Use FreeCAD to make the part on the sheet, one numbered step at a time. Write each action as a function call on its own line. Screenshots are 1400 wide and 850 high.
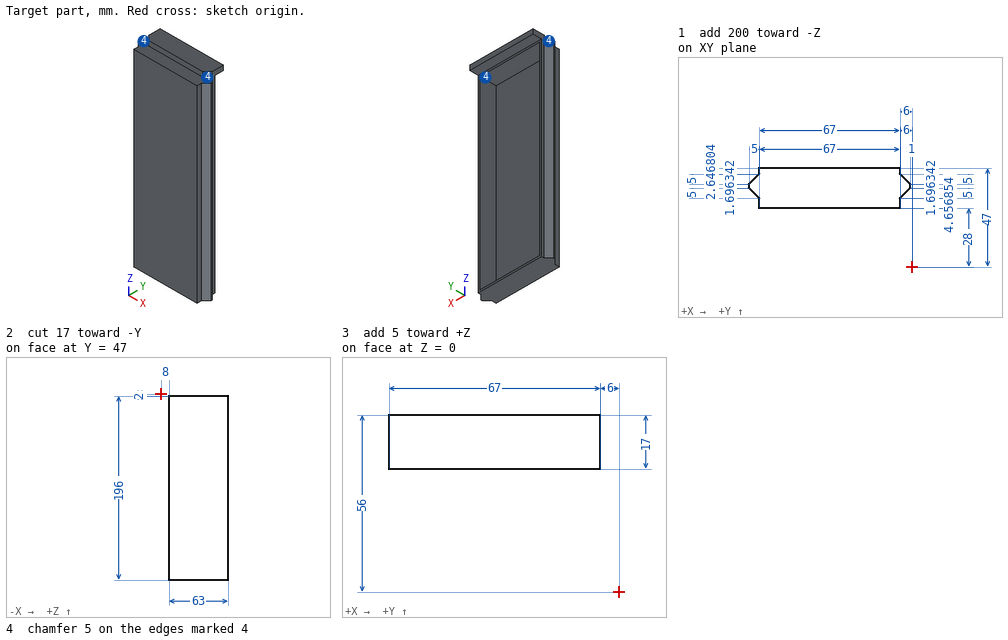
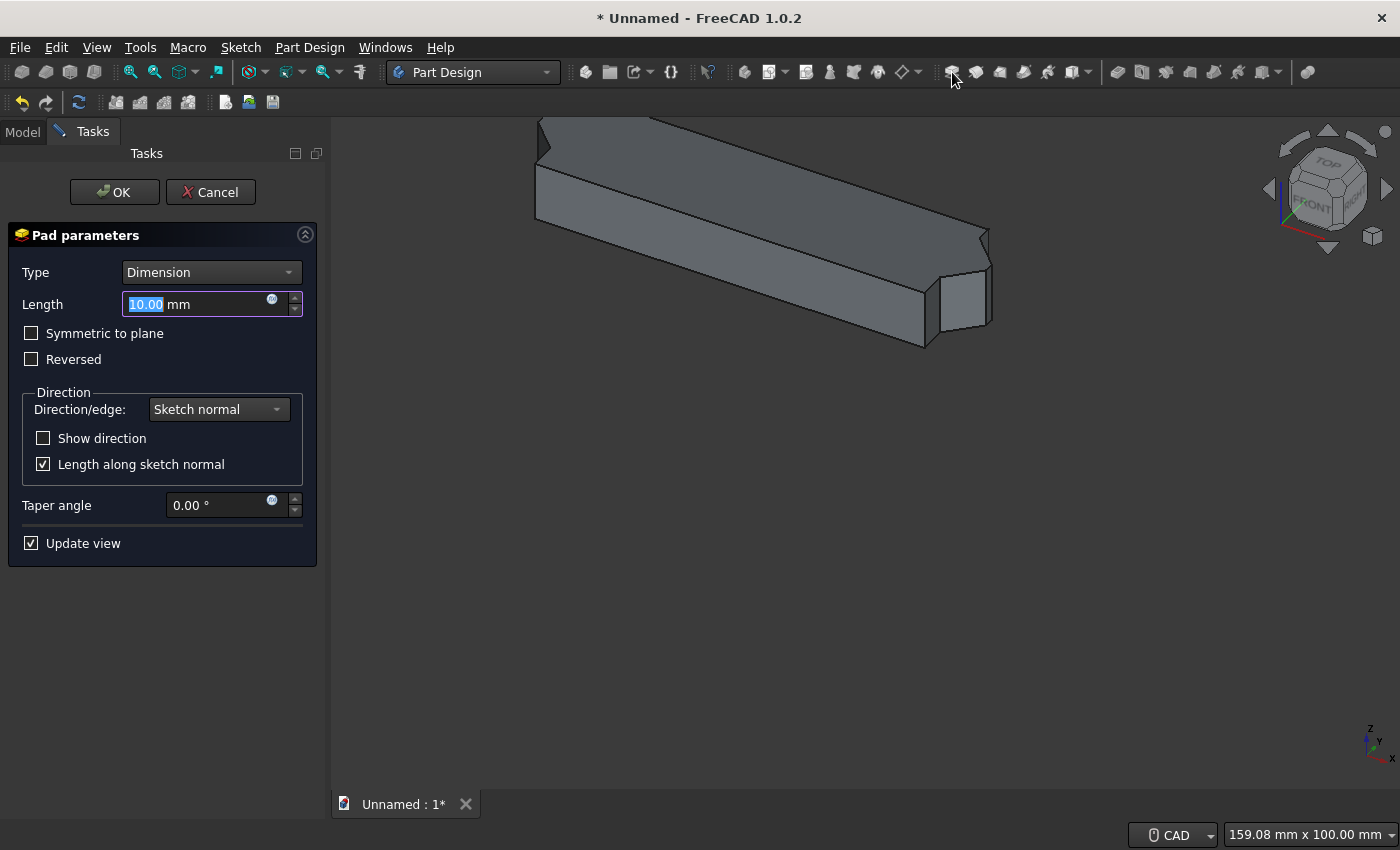
text(200)
key(Tab)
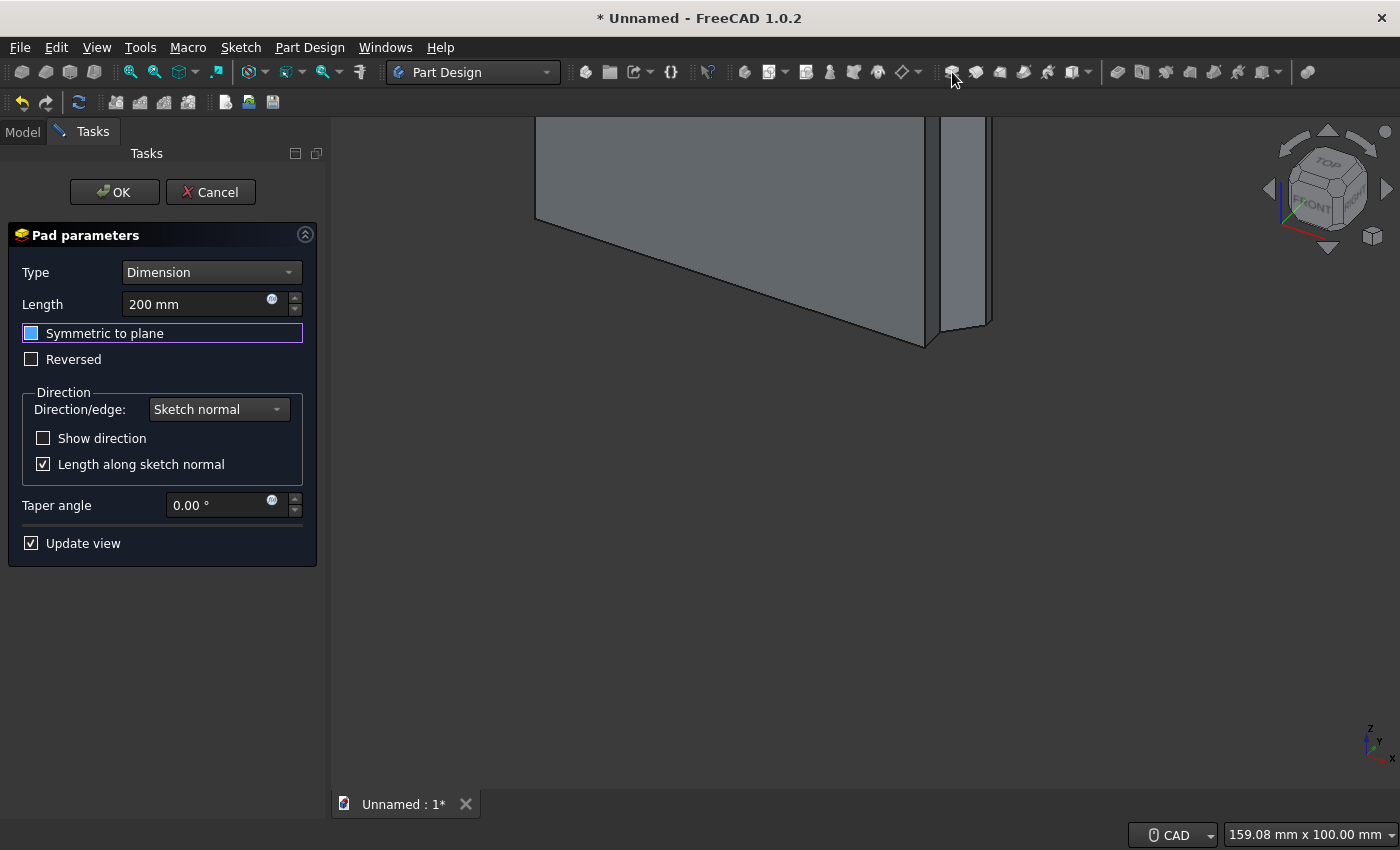
click(30, 359)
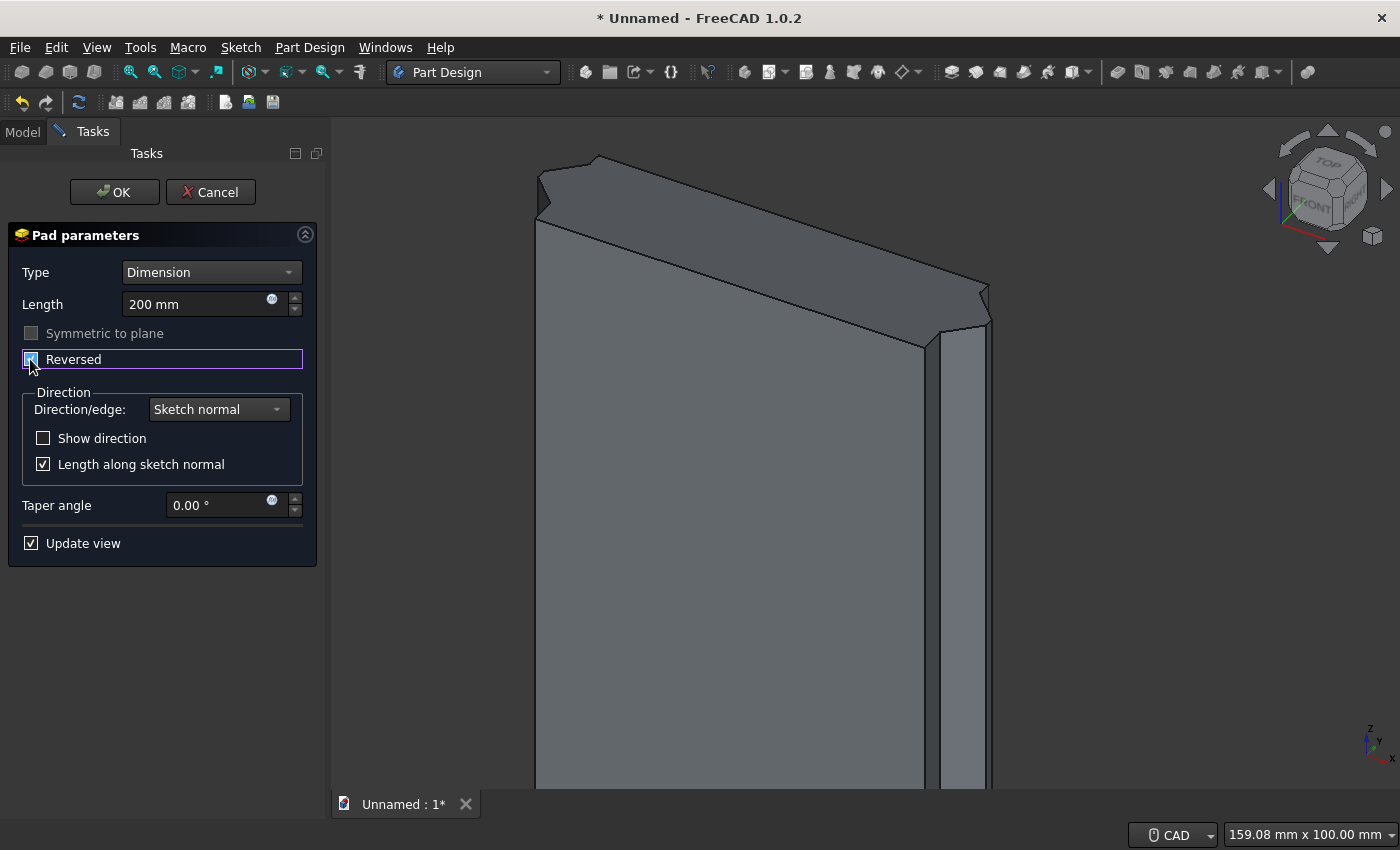
click(115, 192)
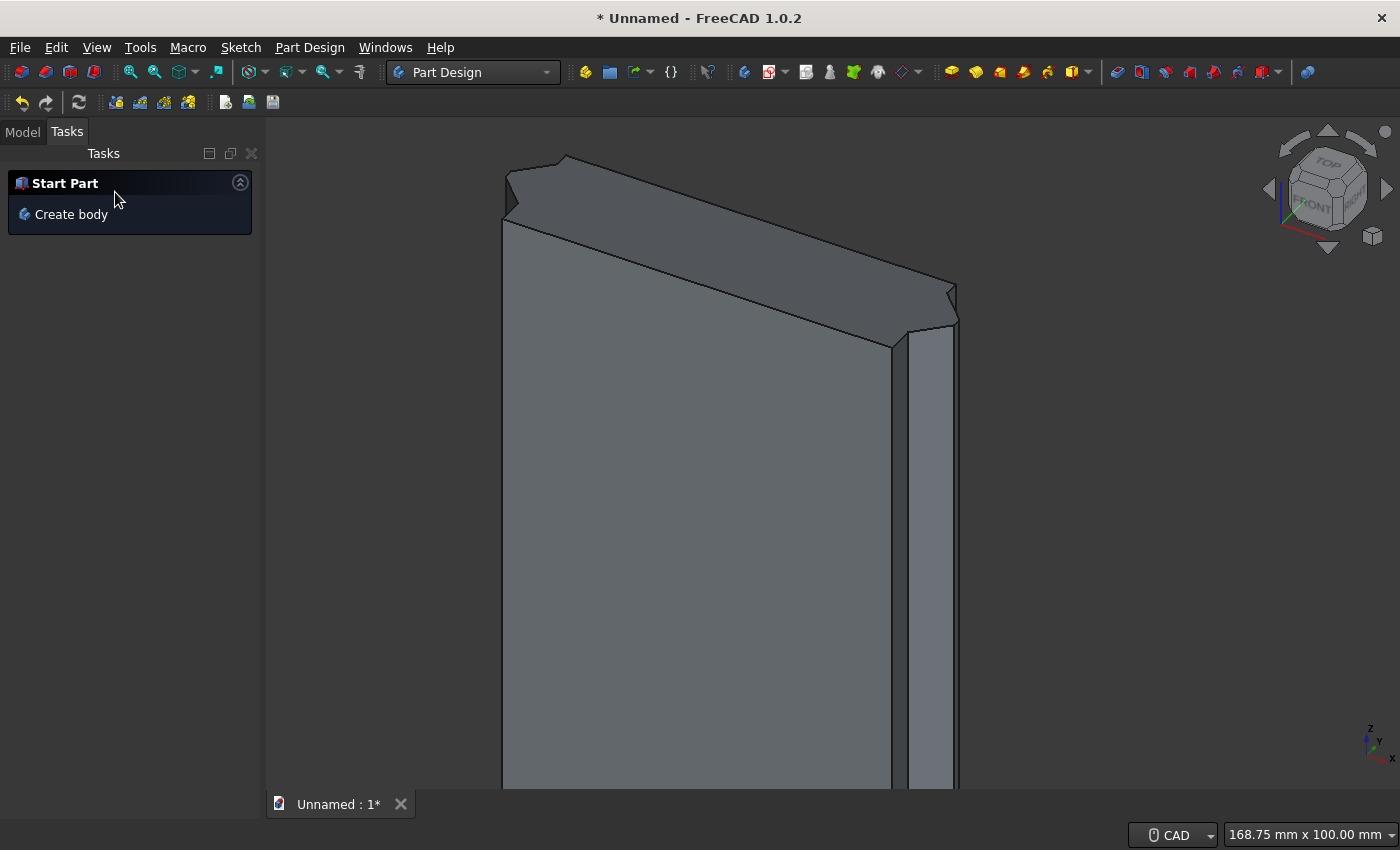
click(132, 72)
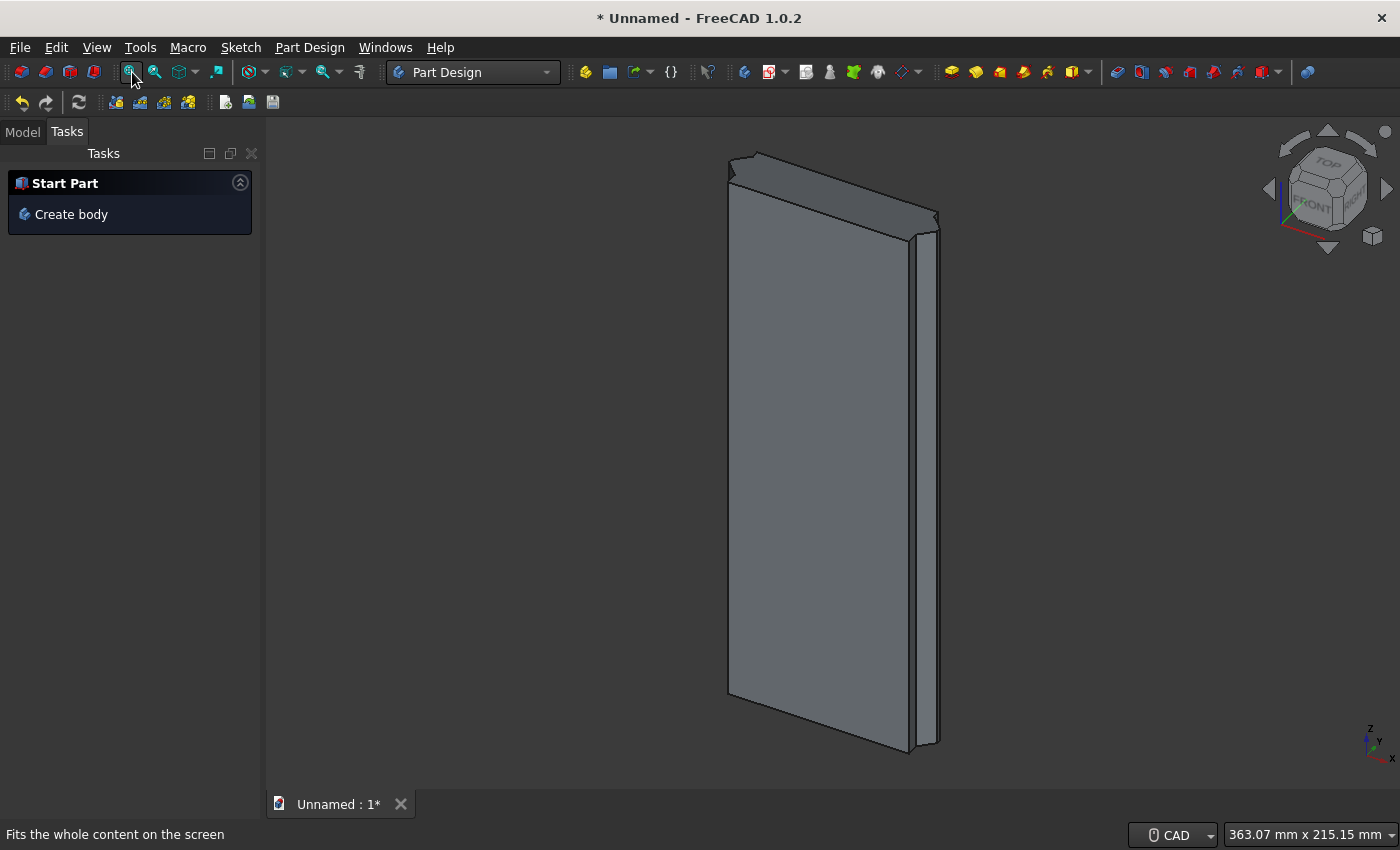
key(4)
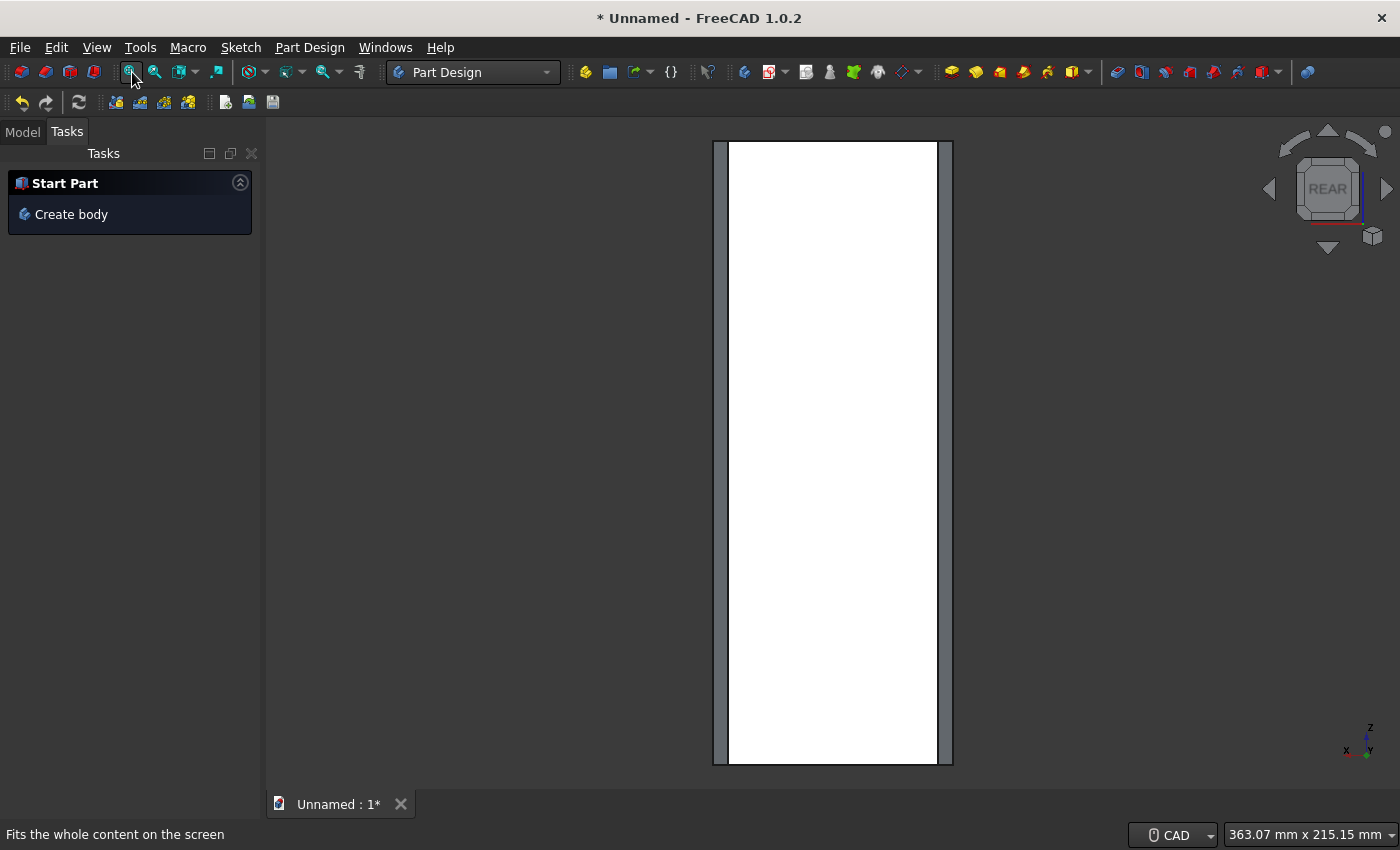
click(833, 274)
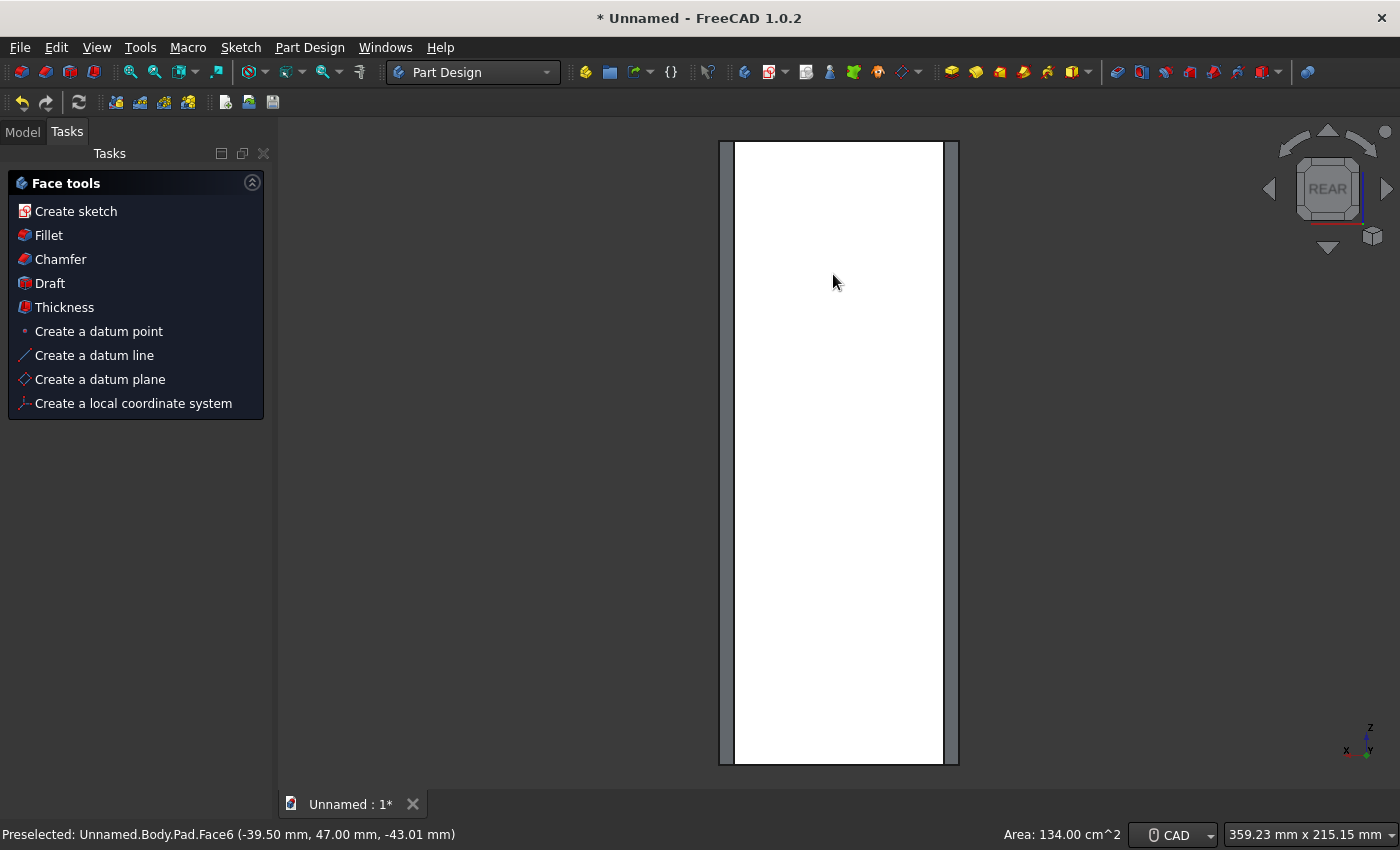
click(770, 72)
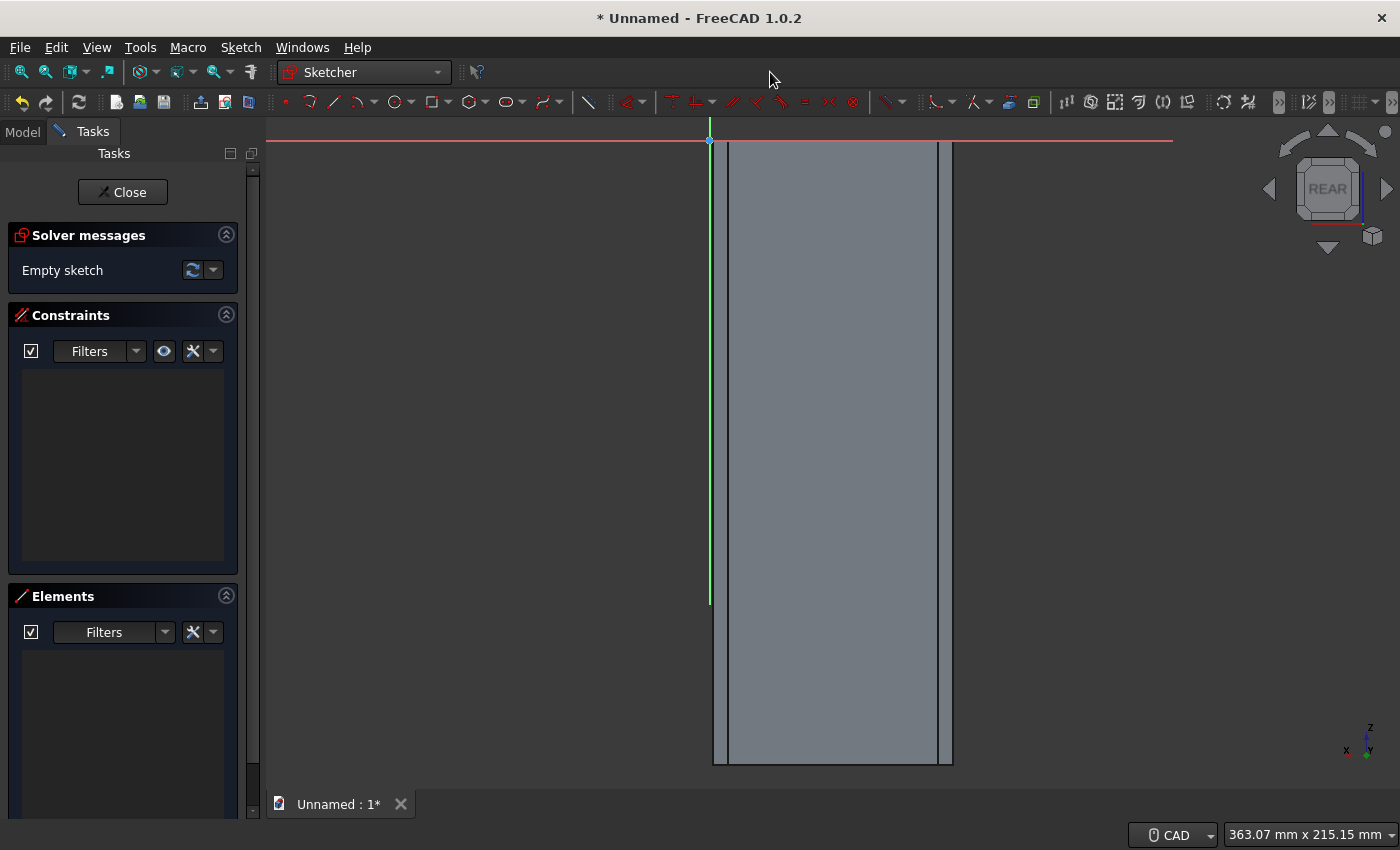
scroll(651, 459, down, 2)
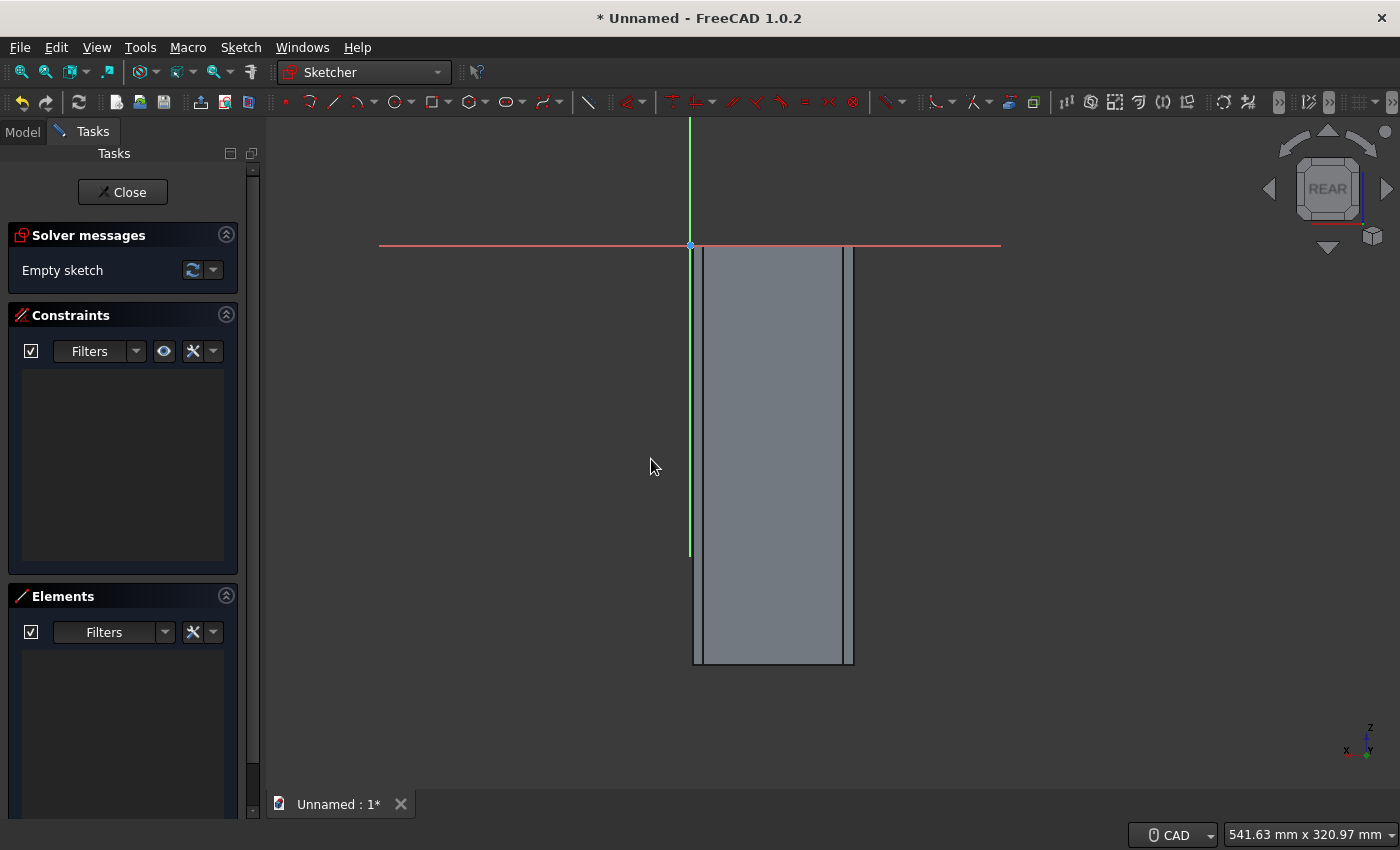
key(g)
key(r)